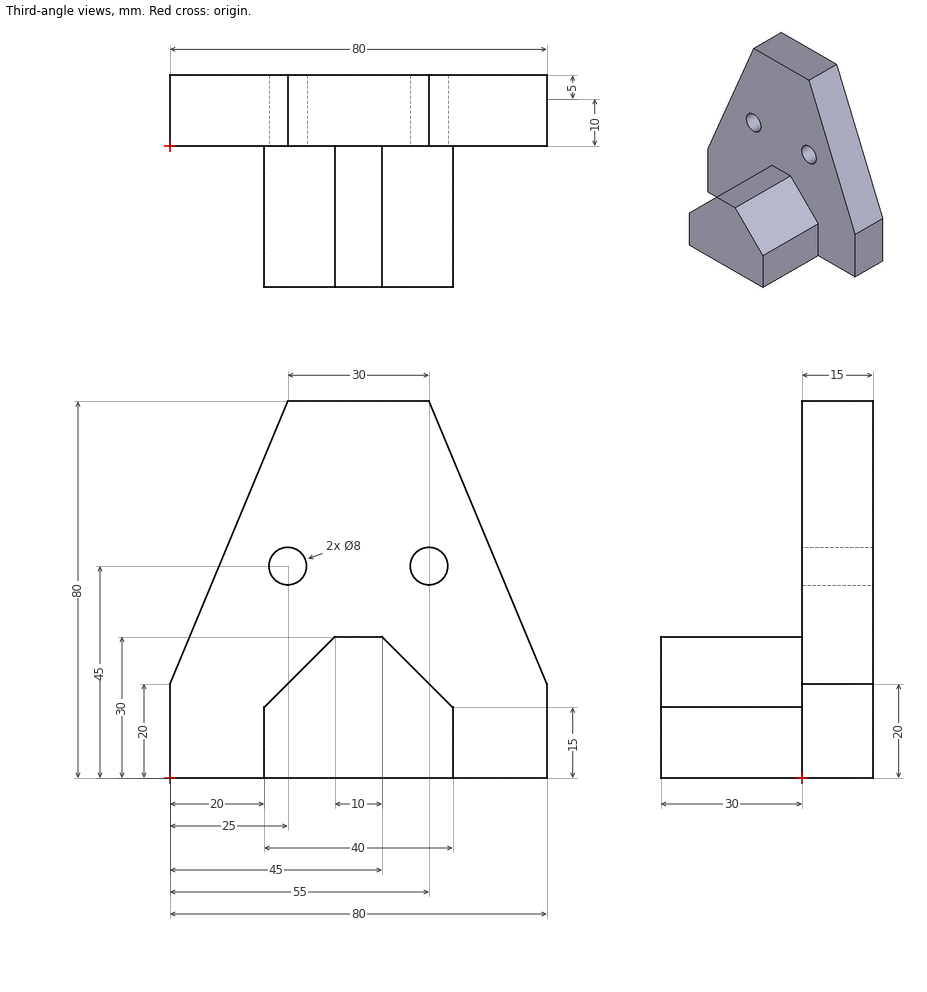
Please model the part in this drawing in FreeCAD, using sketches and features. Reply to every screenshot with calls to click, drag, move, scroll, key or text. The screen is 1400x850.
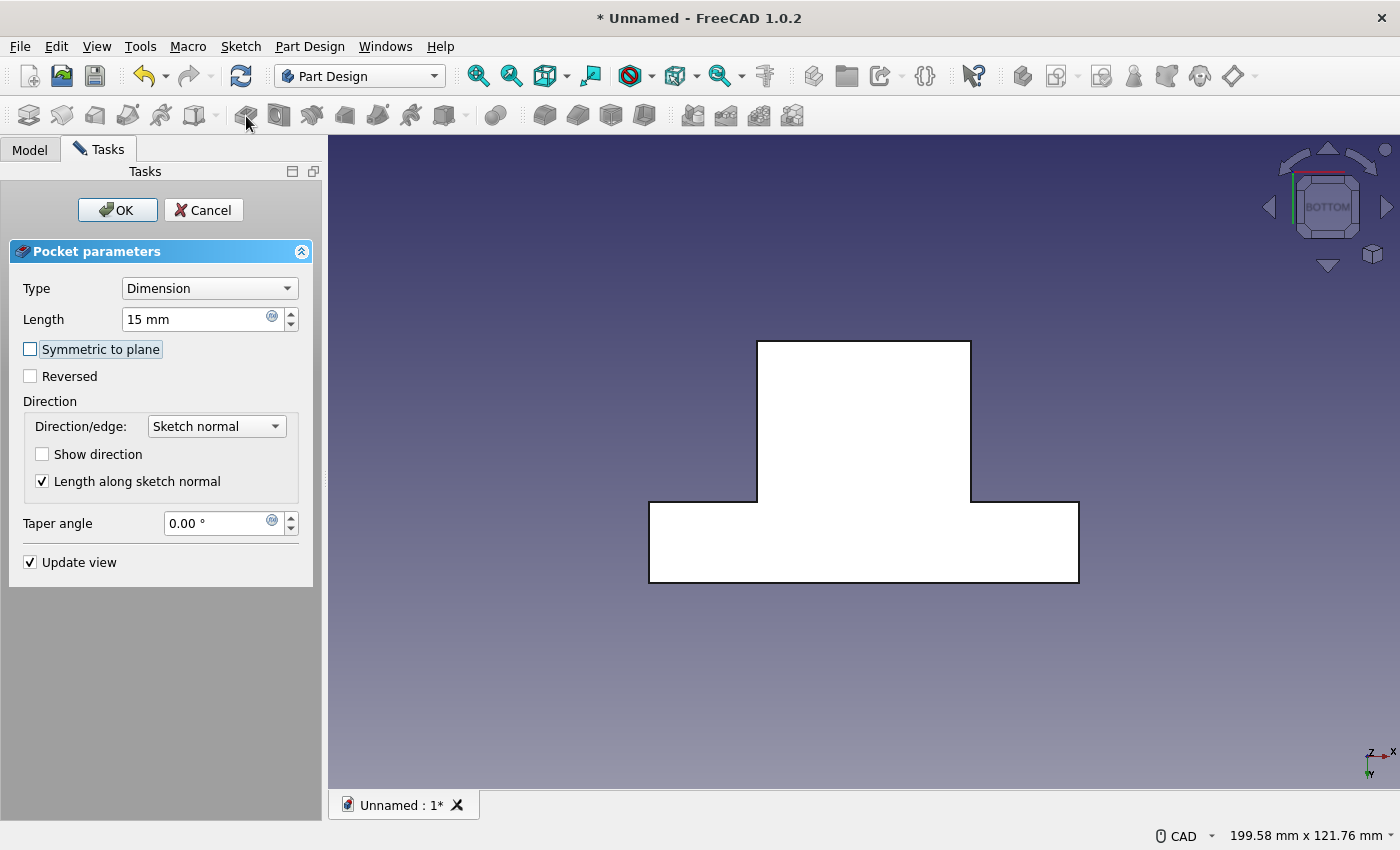
click(118, 210)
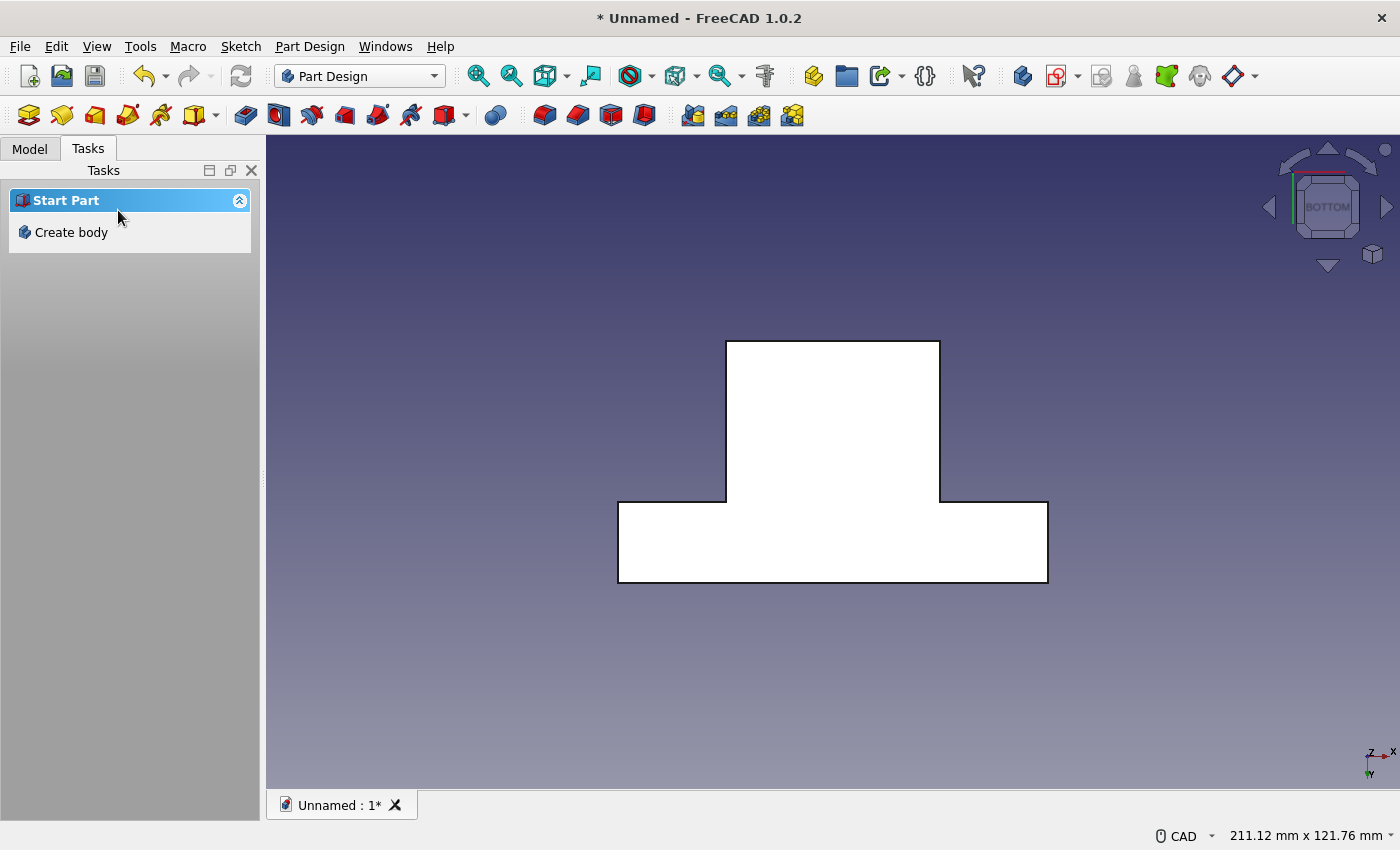
key(0)